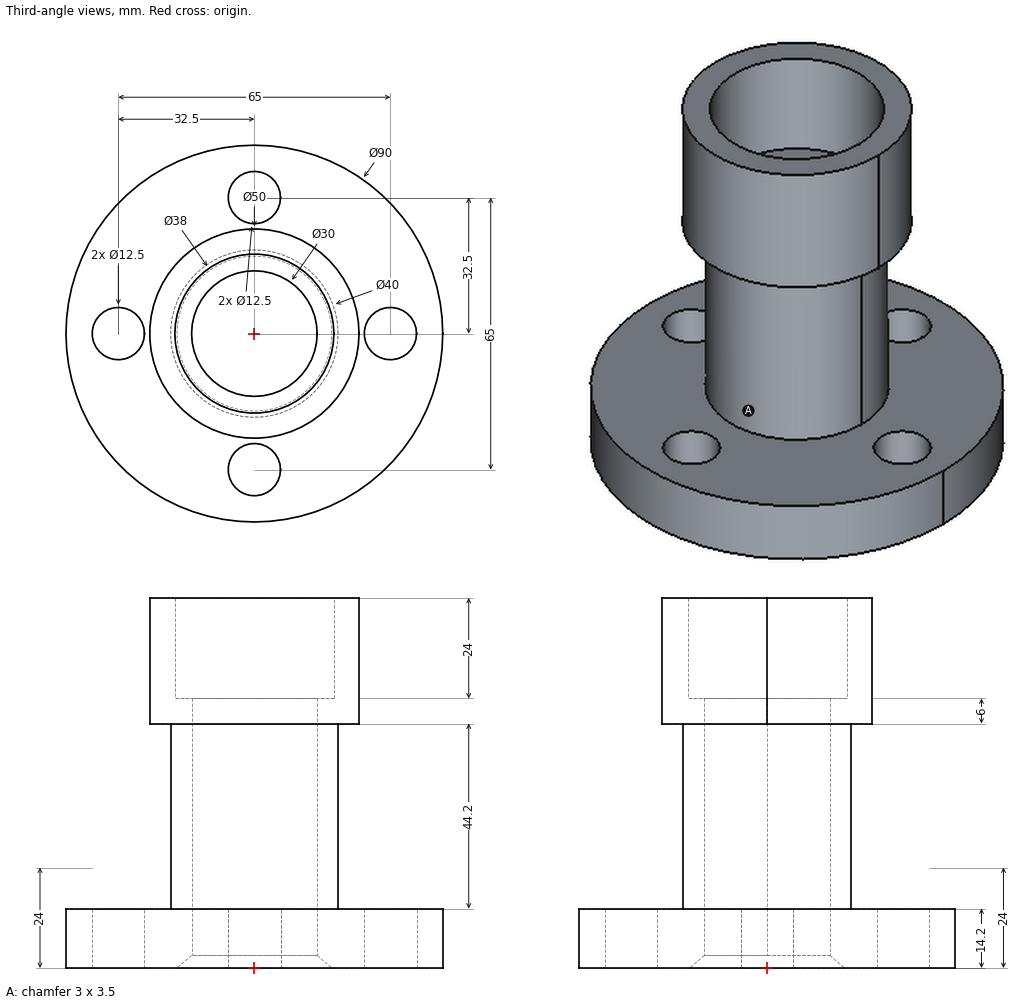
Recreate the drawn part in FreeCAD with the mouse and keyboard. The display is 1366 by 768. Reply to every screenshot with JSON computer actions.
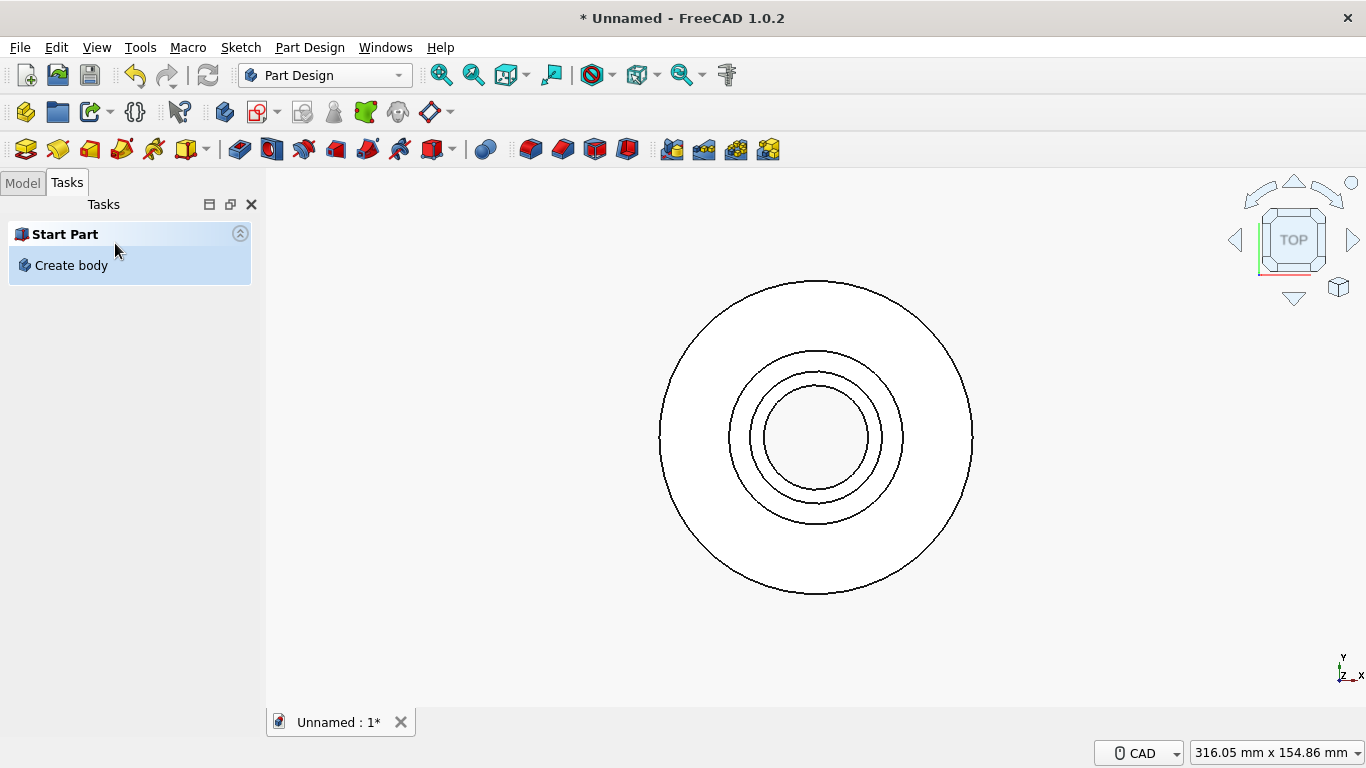
{"action": "key", "text": "1"}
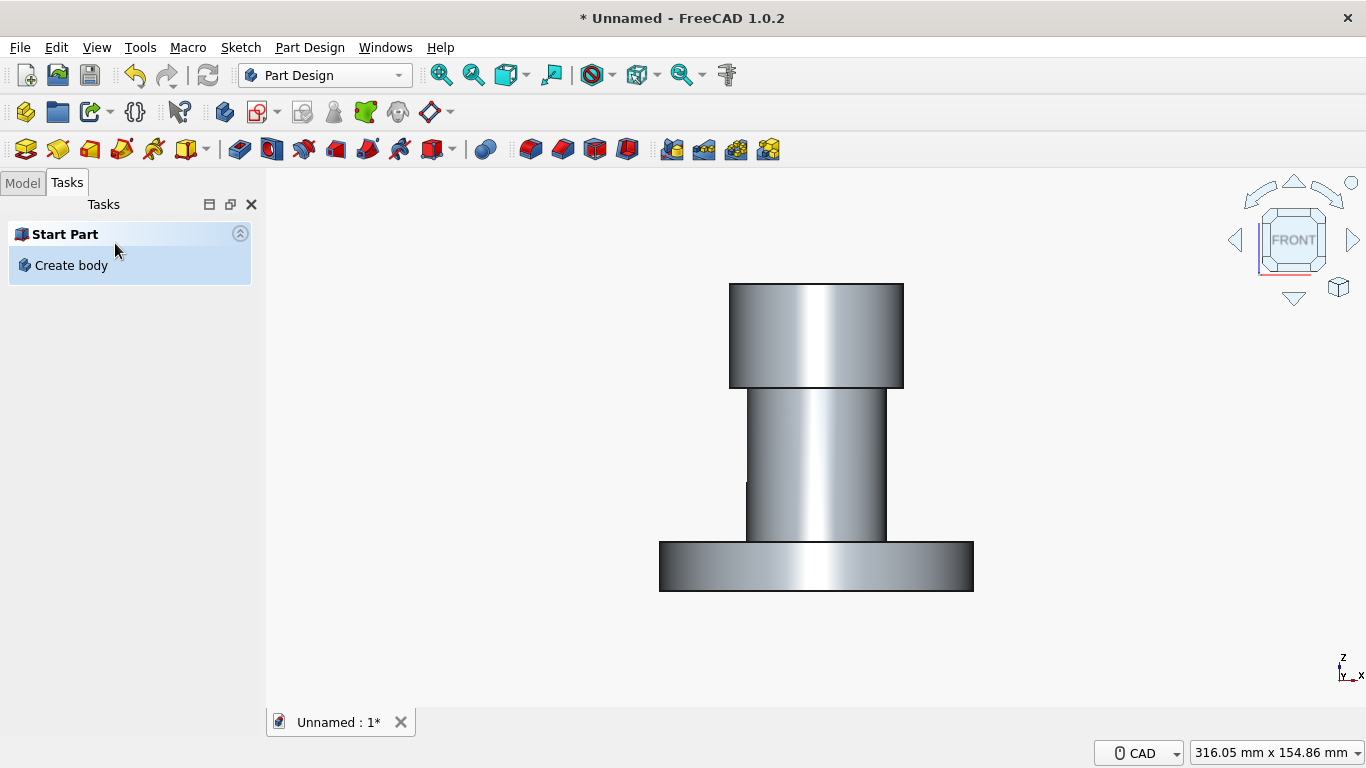
{"action": "key", "text": "3"}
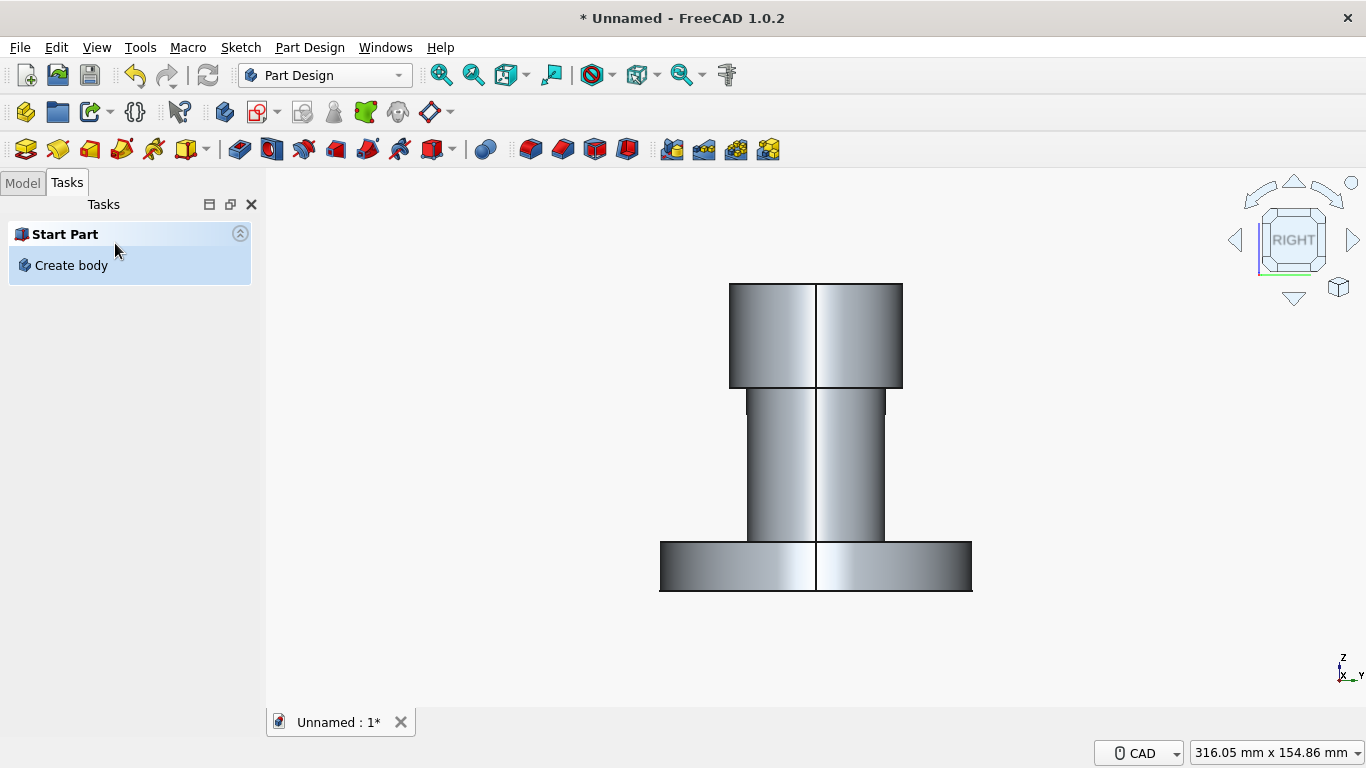
{"action": "key", "text": "5"}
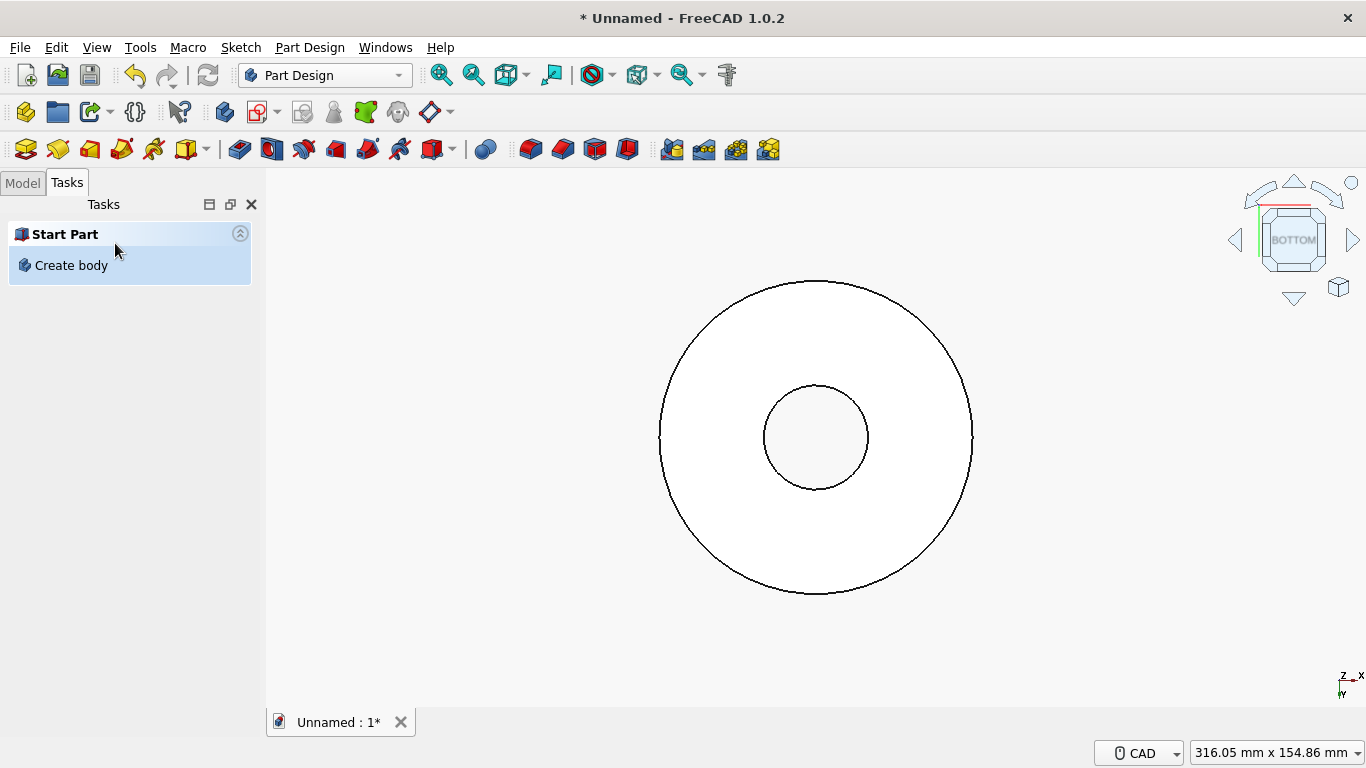
{"action": "left_click", "coordinate": [764, 436]}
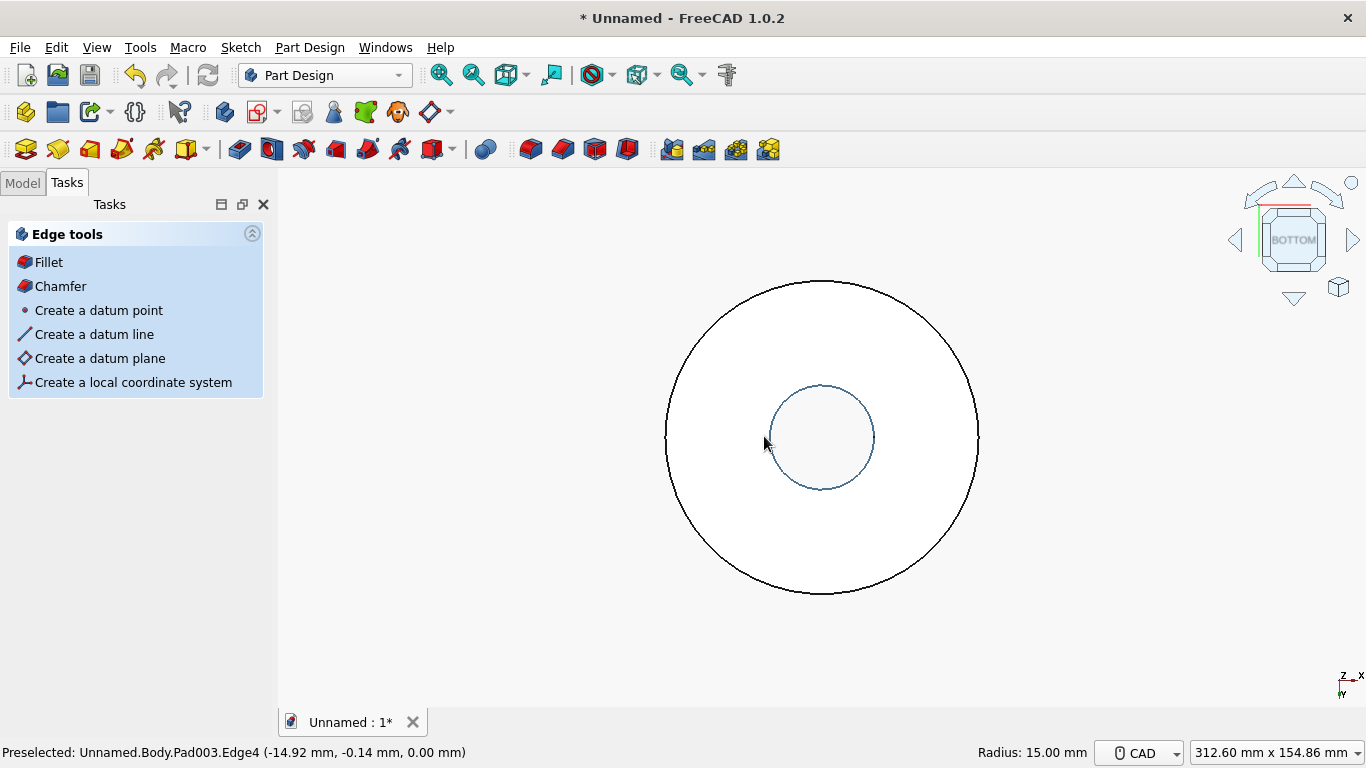
{"action": "left_click", "coordinate": [564, 150]}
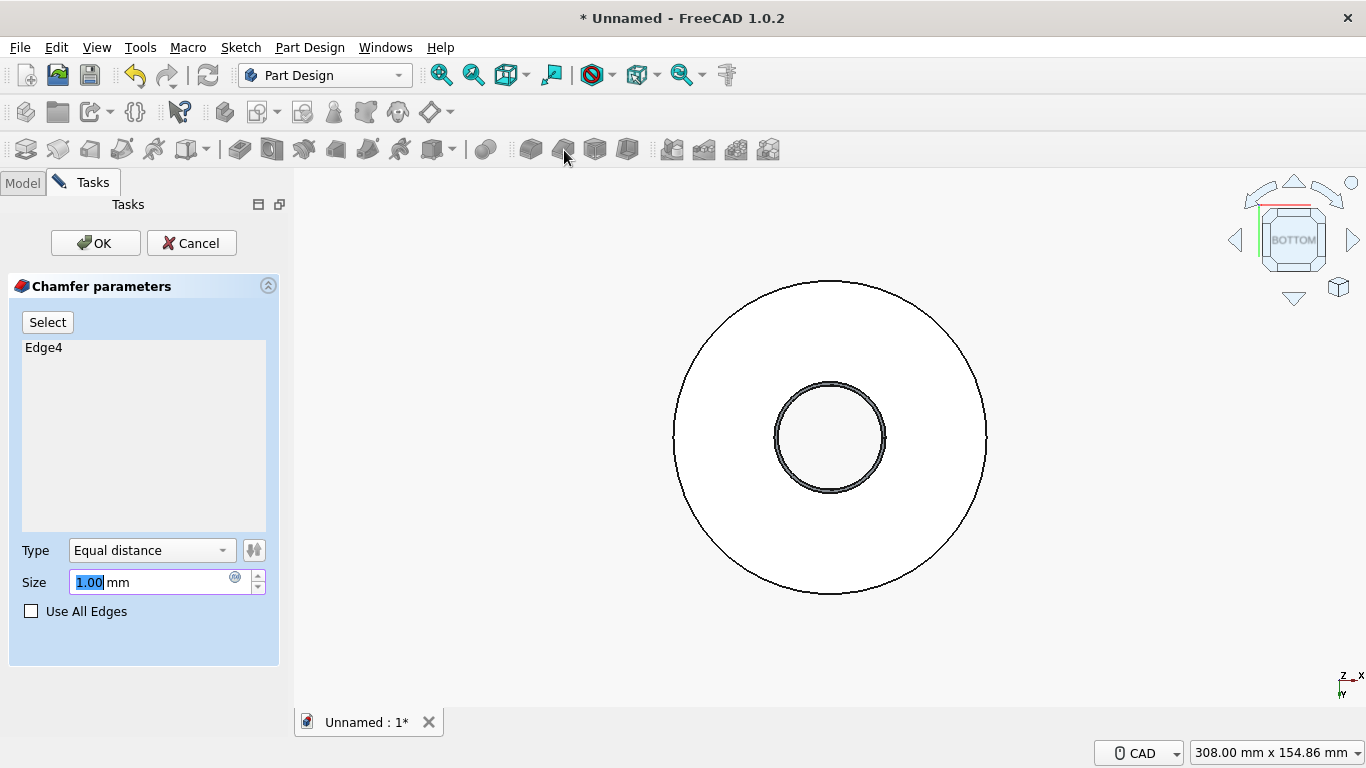
{"action": "type", "text": "3"}
{"action": "key", "text": "Tab"}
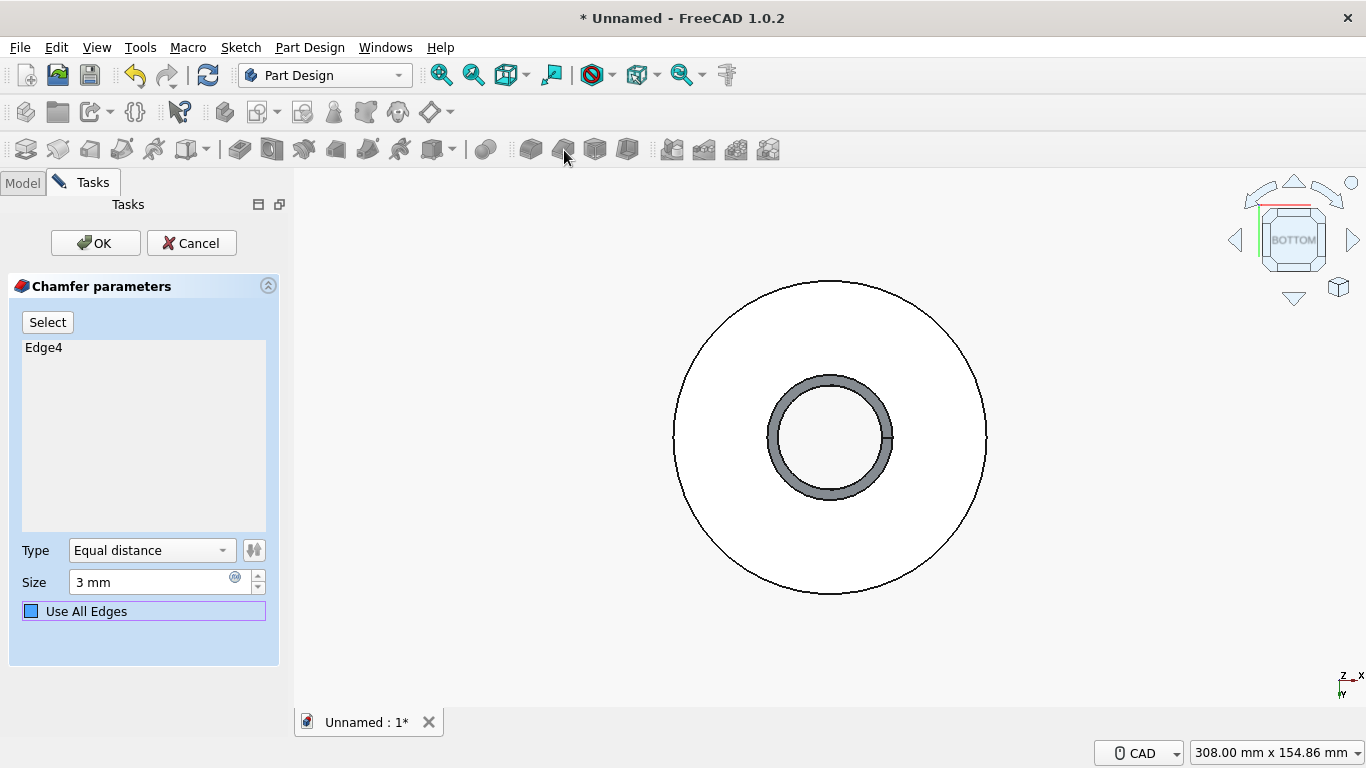
{"action": "left_click", "coordinate": [153, 550]}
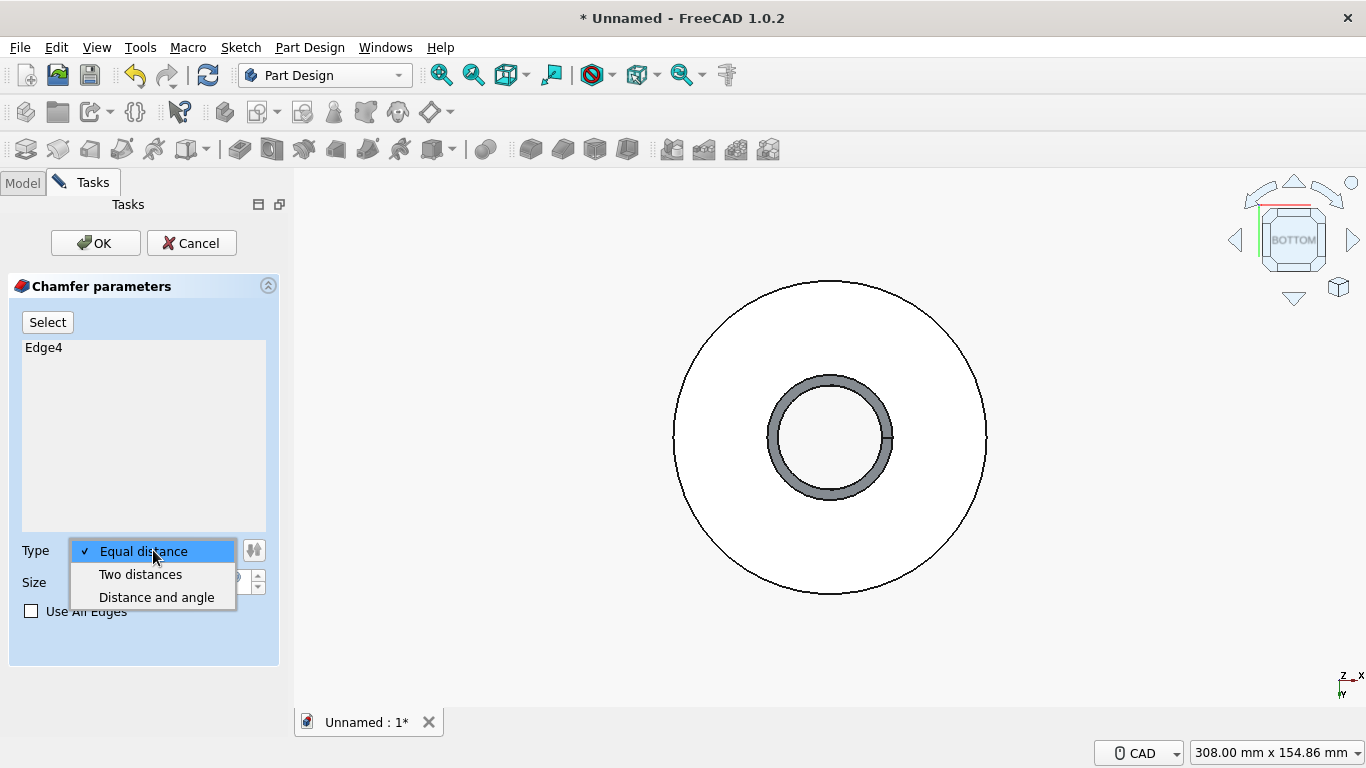
{"action": "left_click", "coordinate": [152, 574]}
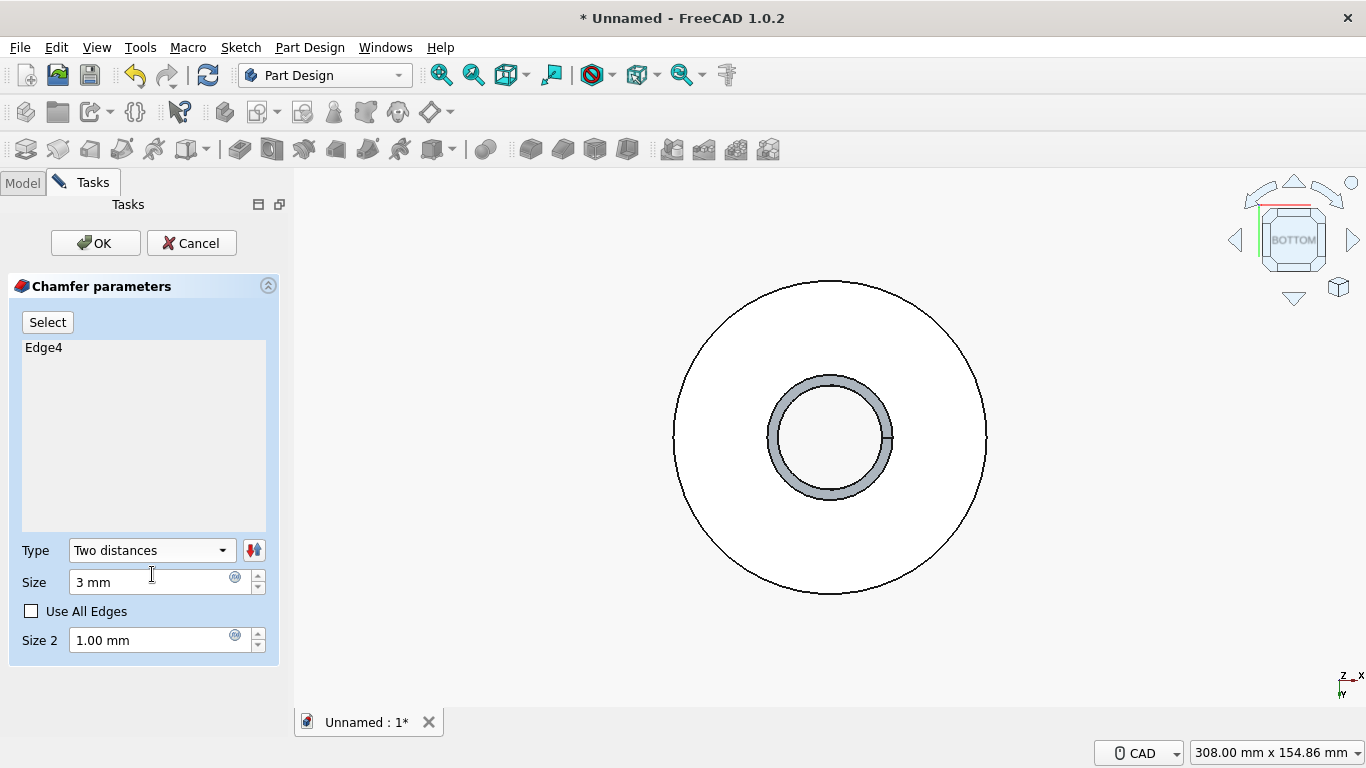
{"action": "triple_click", "coordinate": [160, 640]}